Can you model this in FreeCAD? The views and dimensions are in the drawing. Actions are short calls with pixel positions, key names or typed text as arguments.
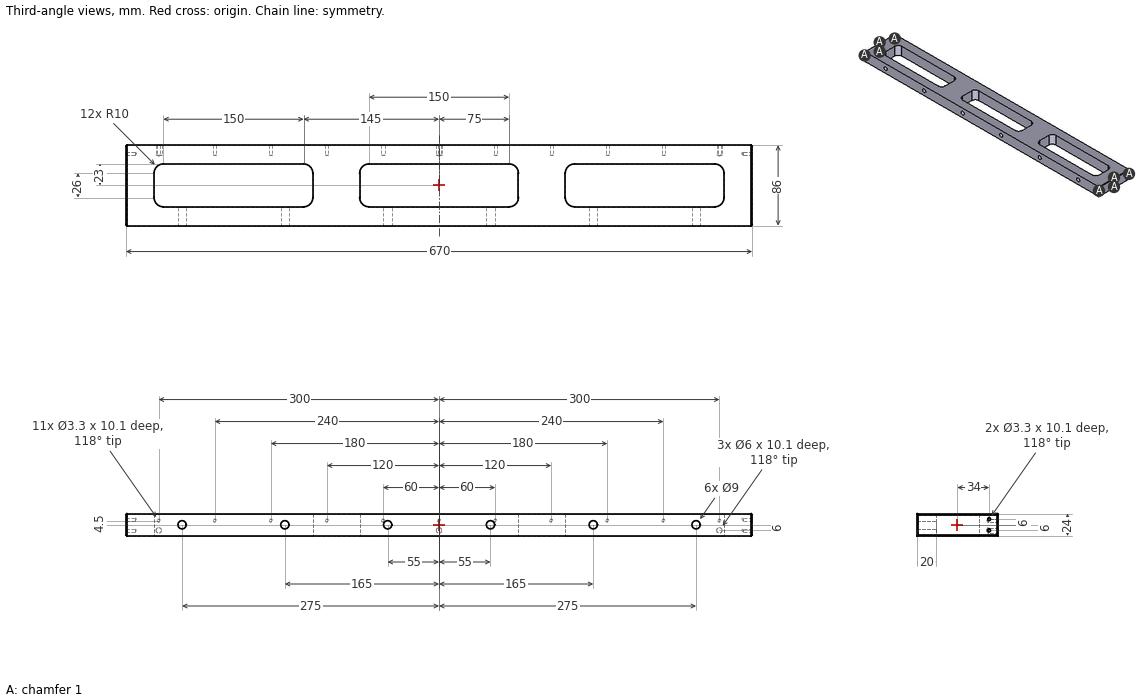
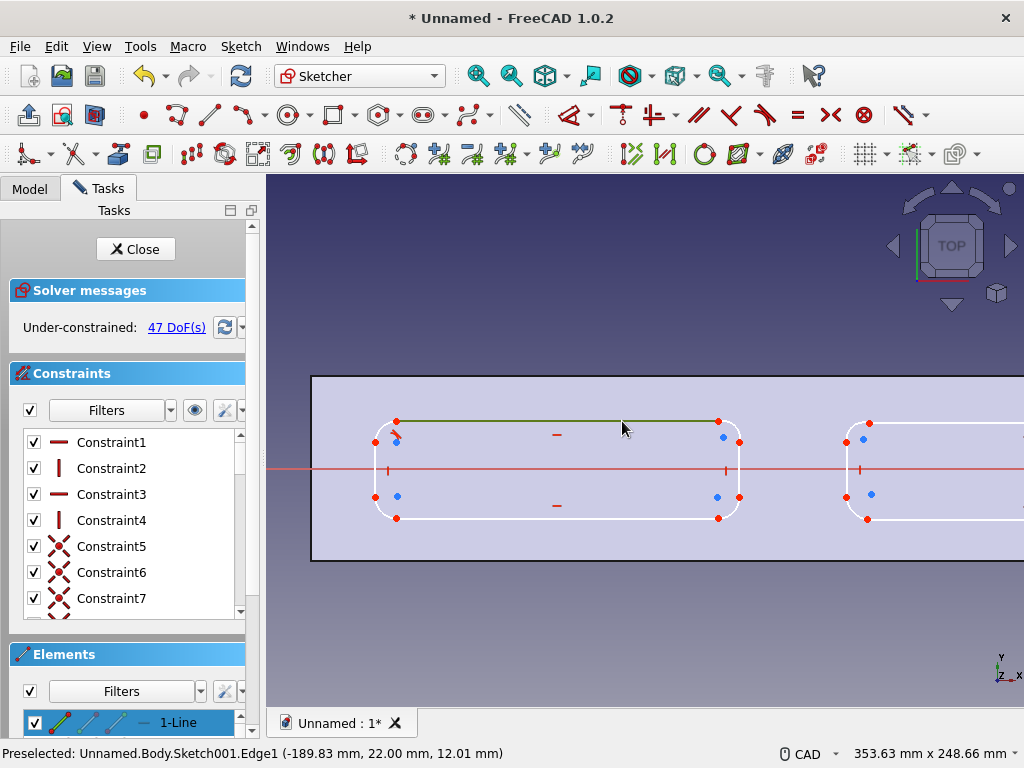
scroll(739, 432, up, 2)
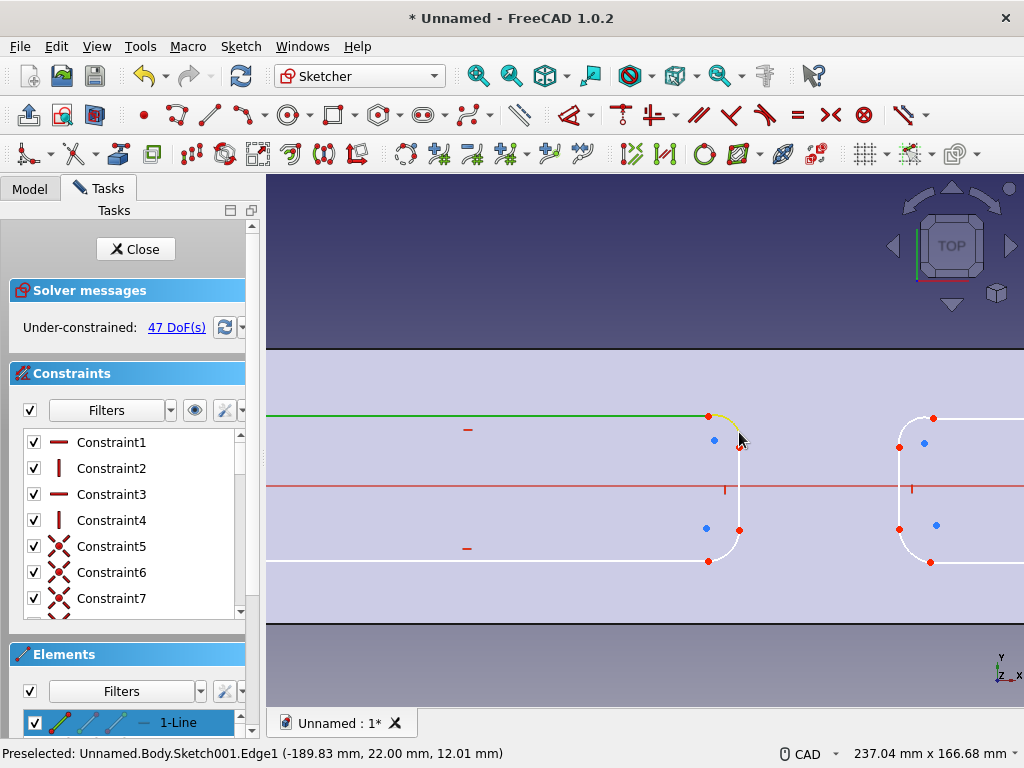
click(739, 432)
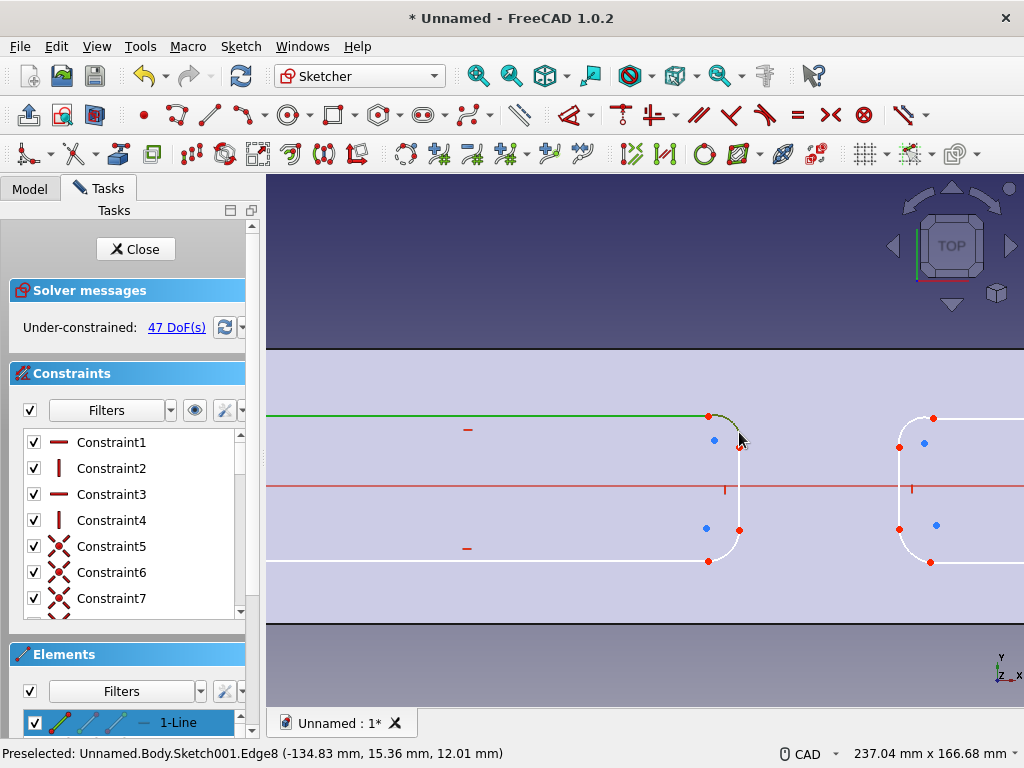
click(765, 116)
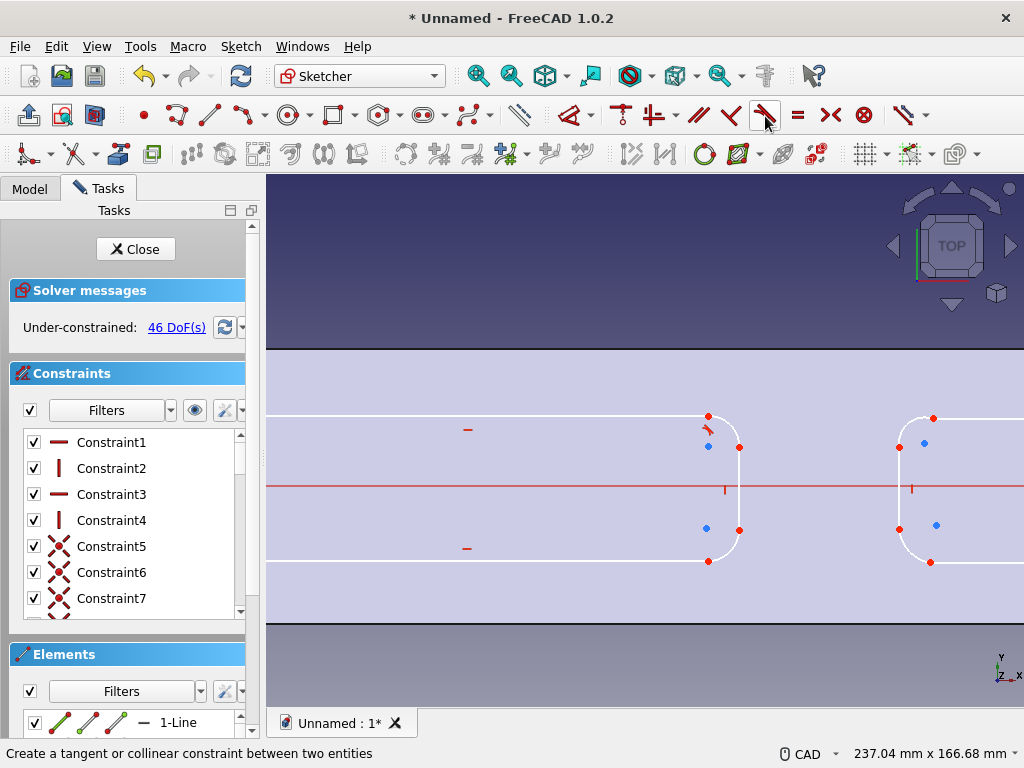
scroll(426, 429, down, 8)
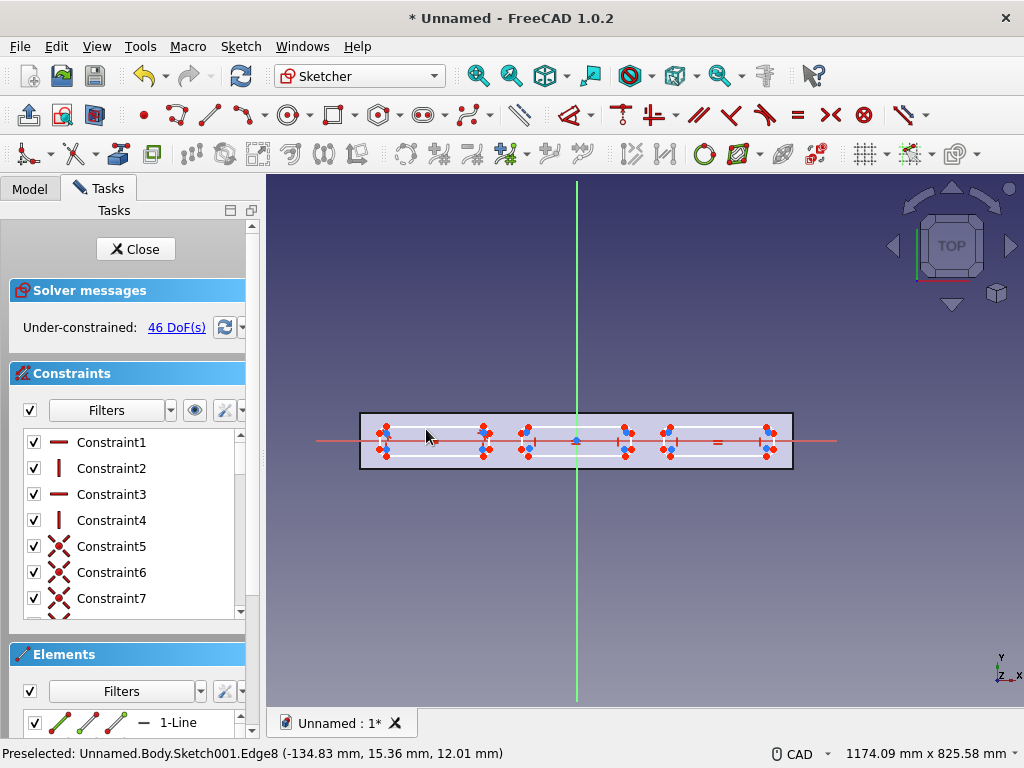
scroll(380, 438, up, 8)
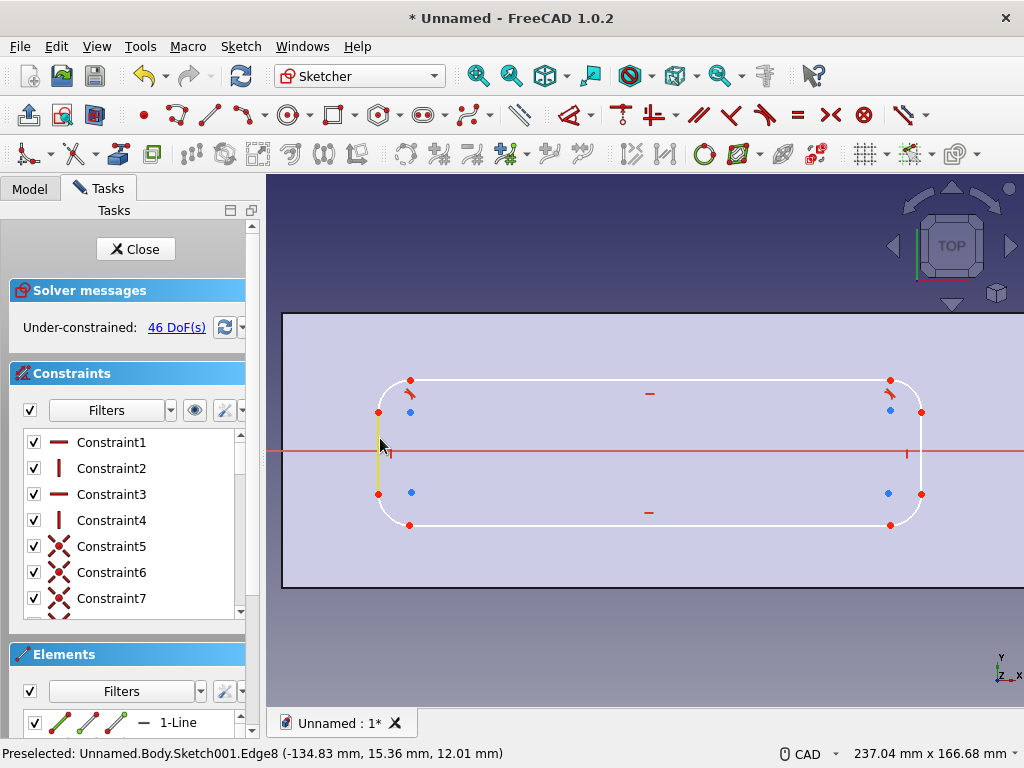
click(378, 437)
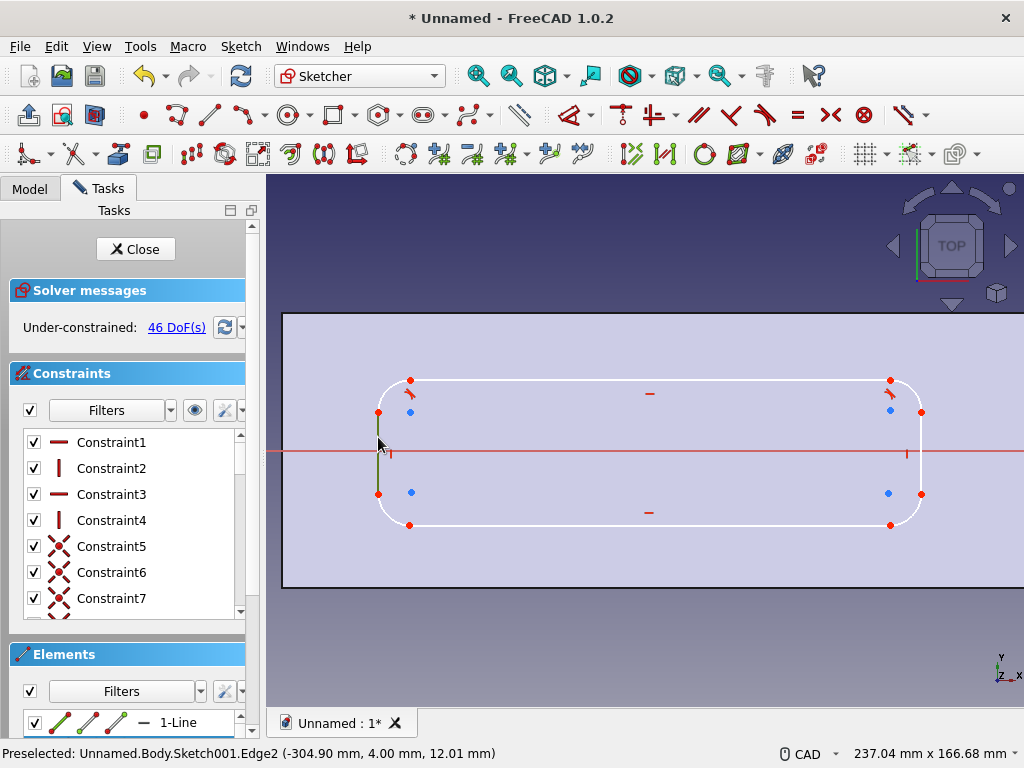
click(396, 384)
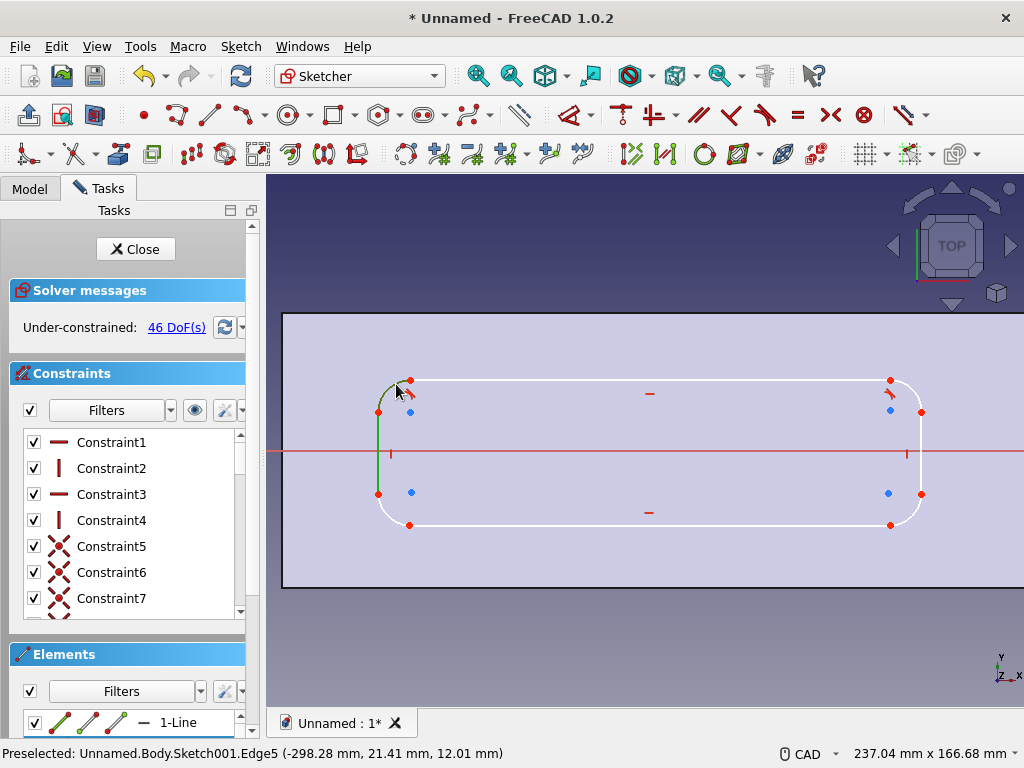
key(t)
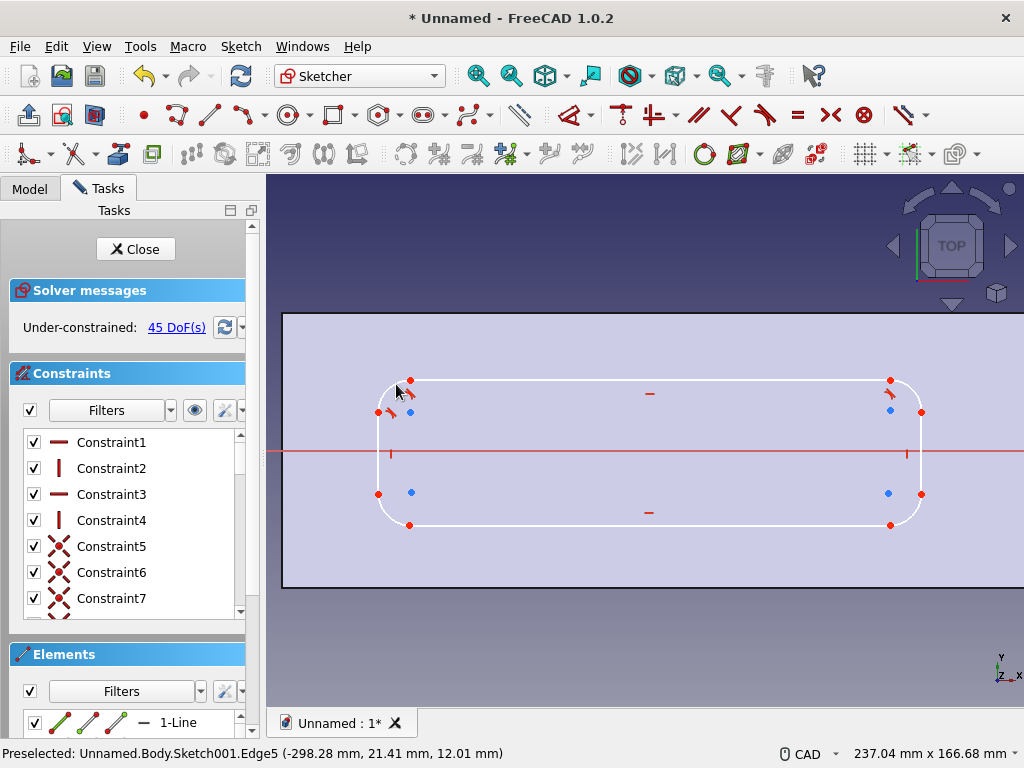
click(378, 437)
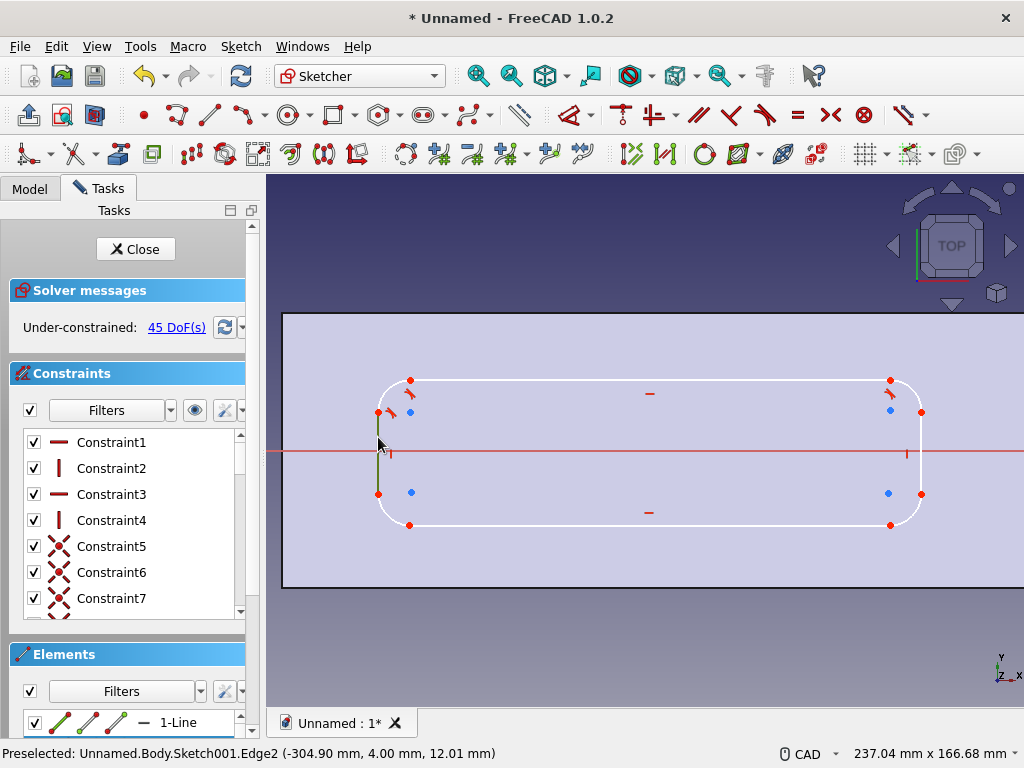
click(382, 508)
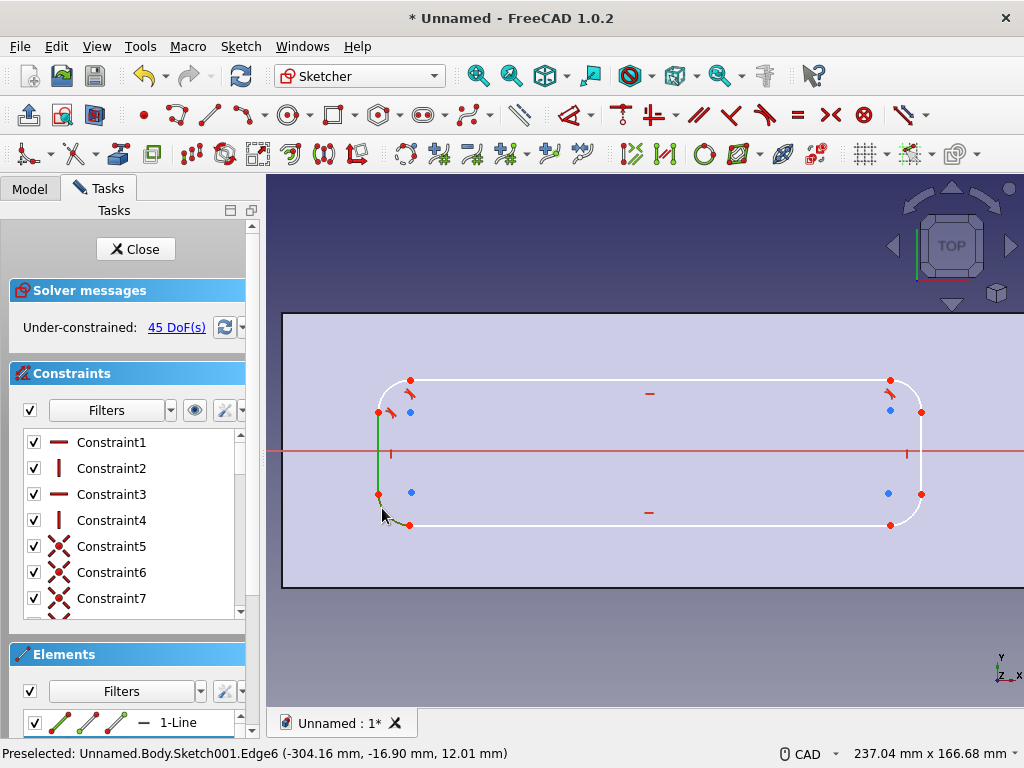
key(t)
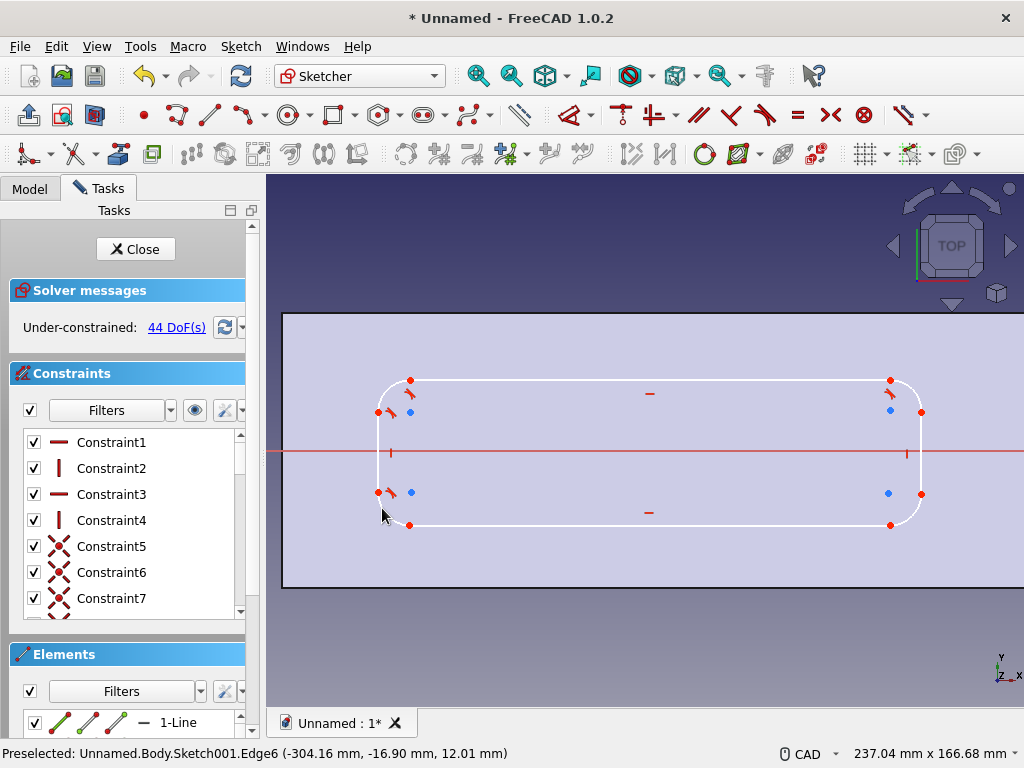
scroll(380, 438, down, 8)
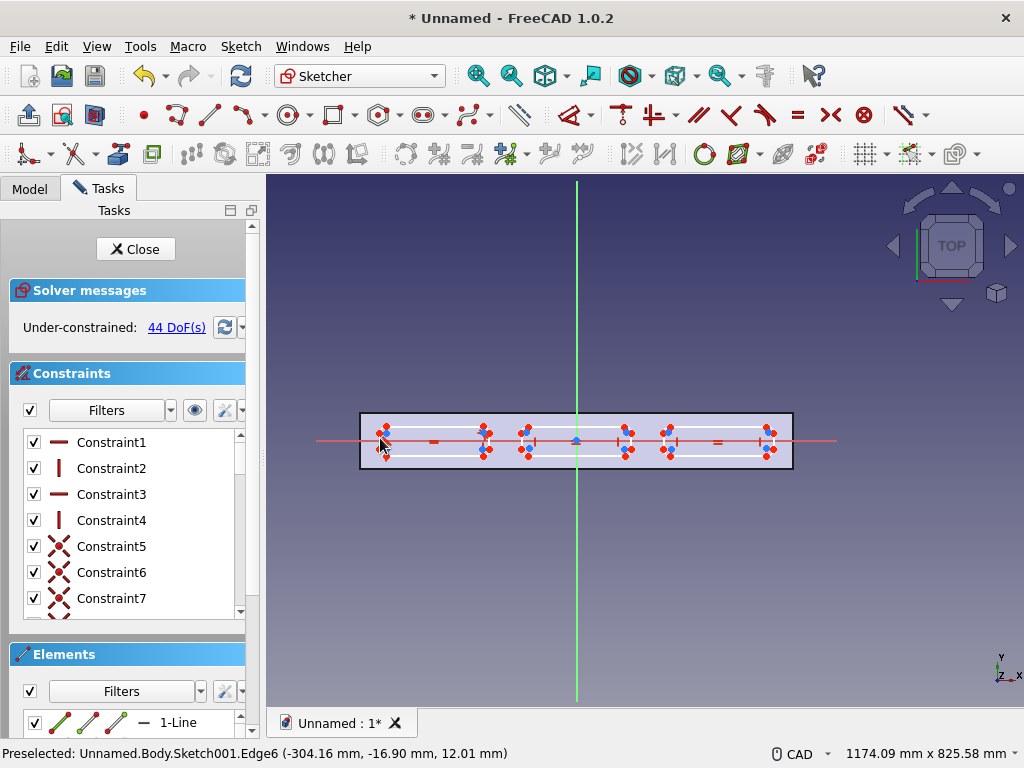
click(415, 456)